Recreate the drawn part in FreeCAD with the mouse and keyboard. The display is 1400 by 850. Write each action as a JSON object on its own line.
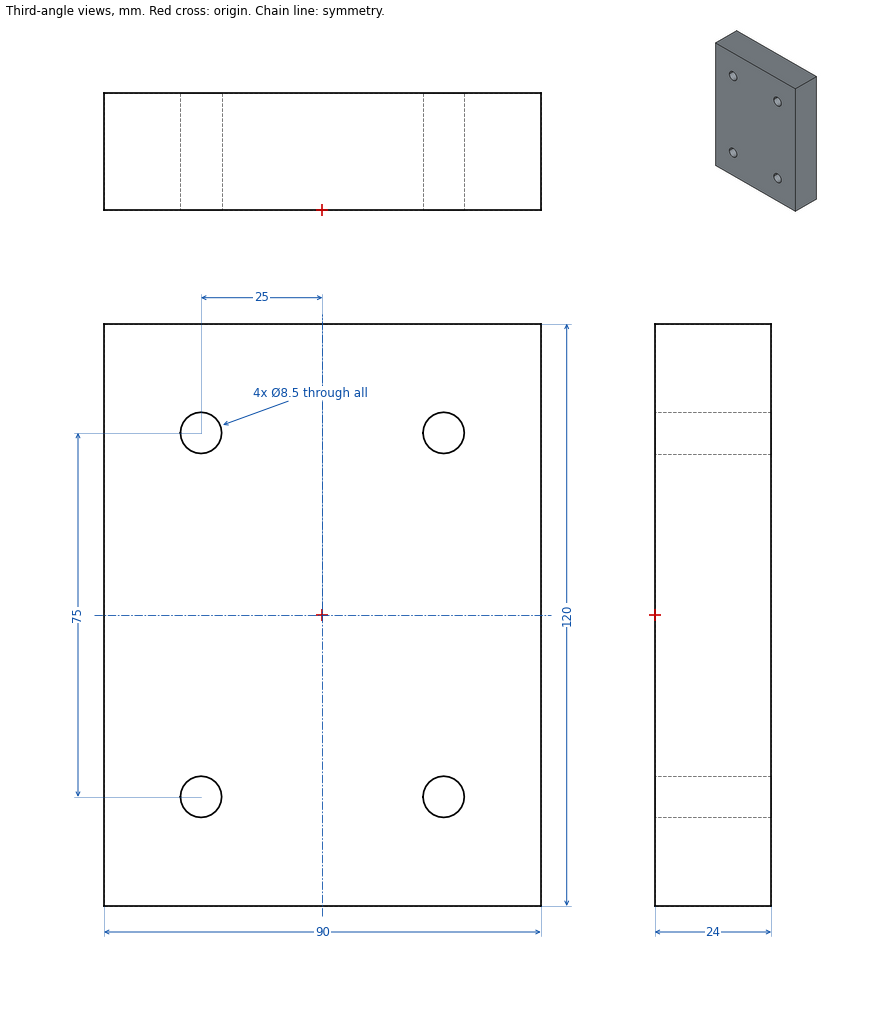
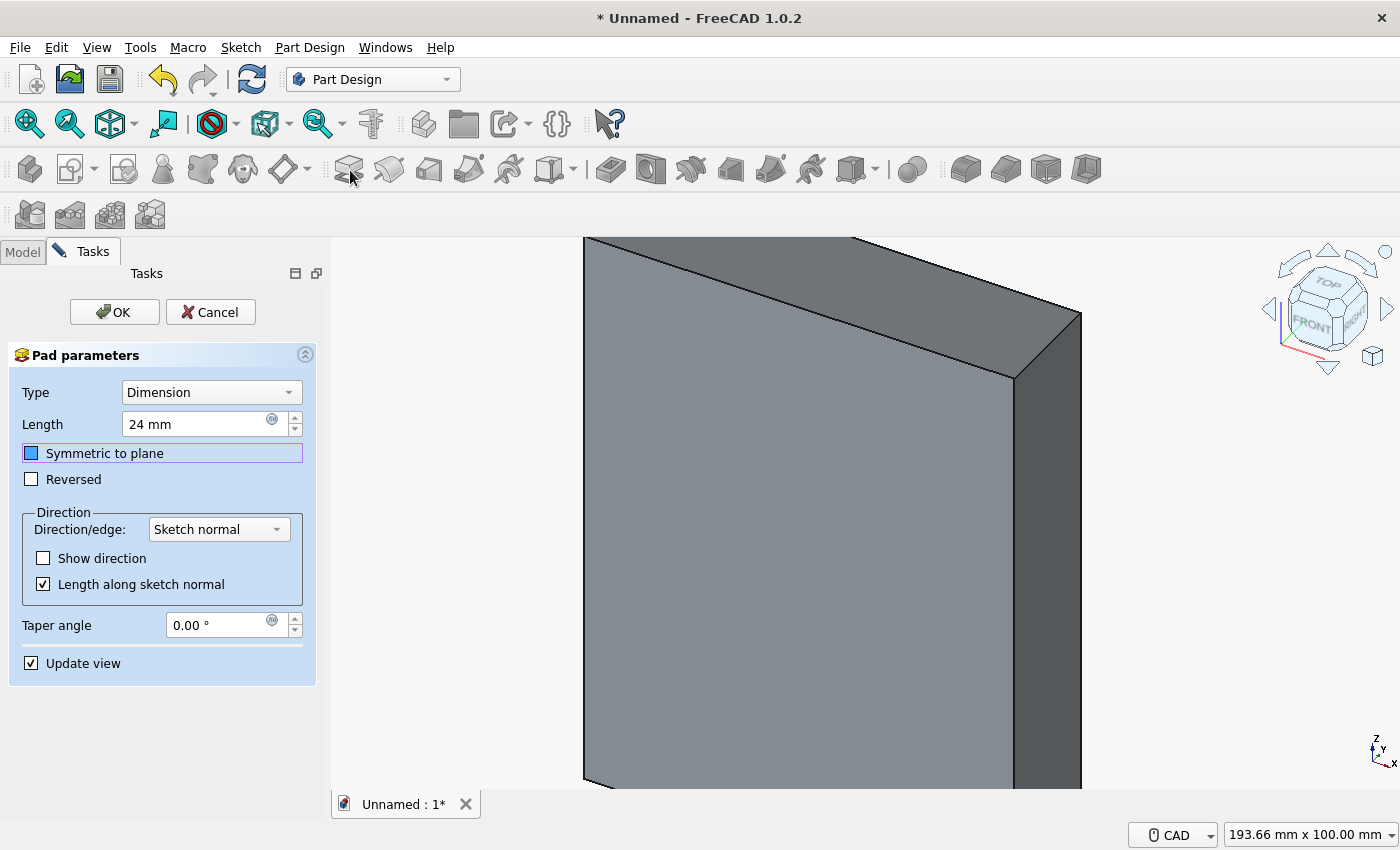
{"action": "left_click", "coordinate": [30, 479]}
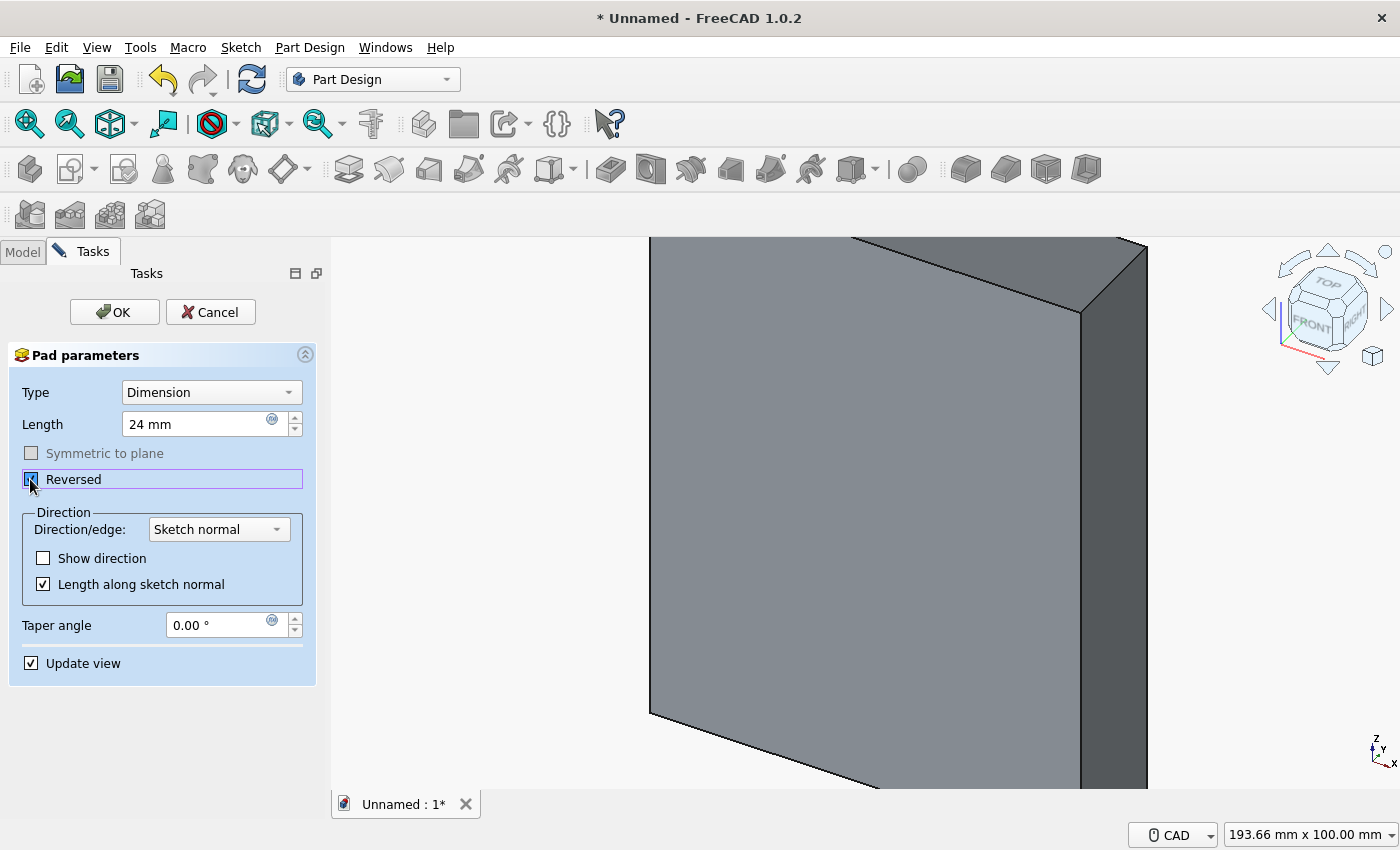
{"action": "left_click", "coordinate": [115, 312]}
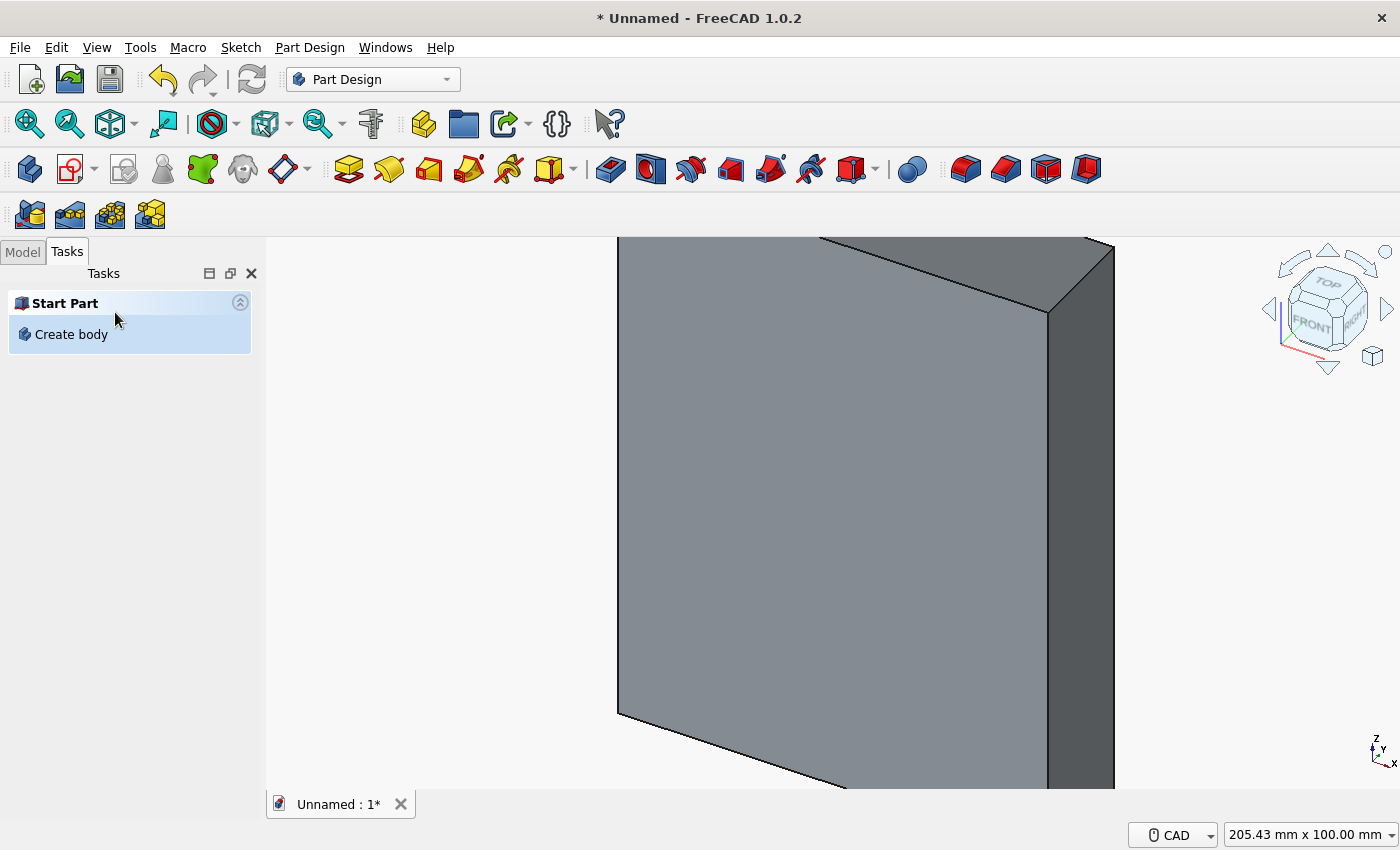
{"action": "left_click", "coordinate": [30, 124]}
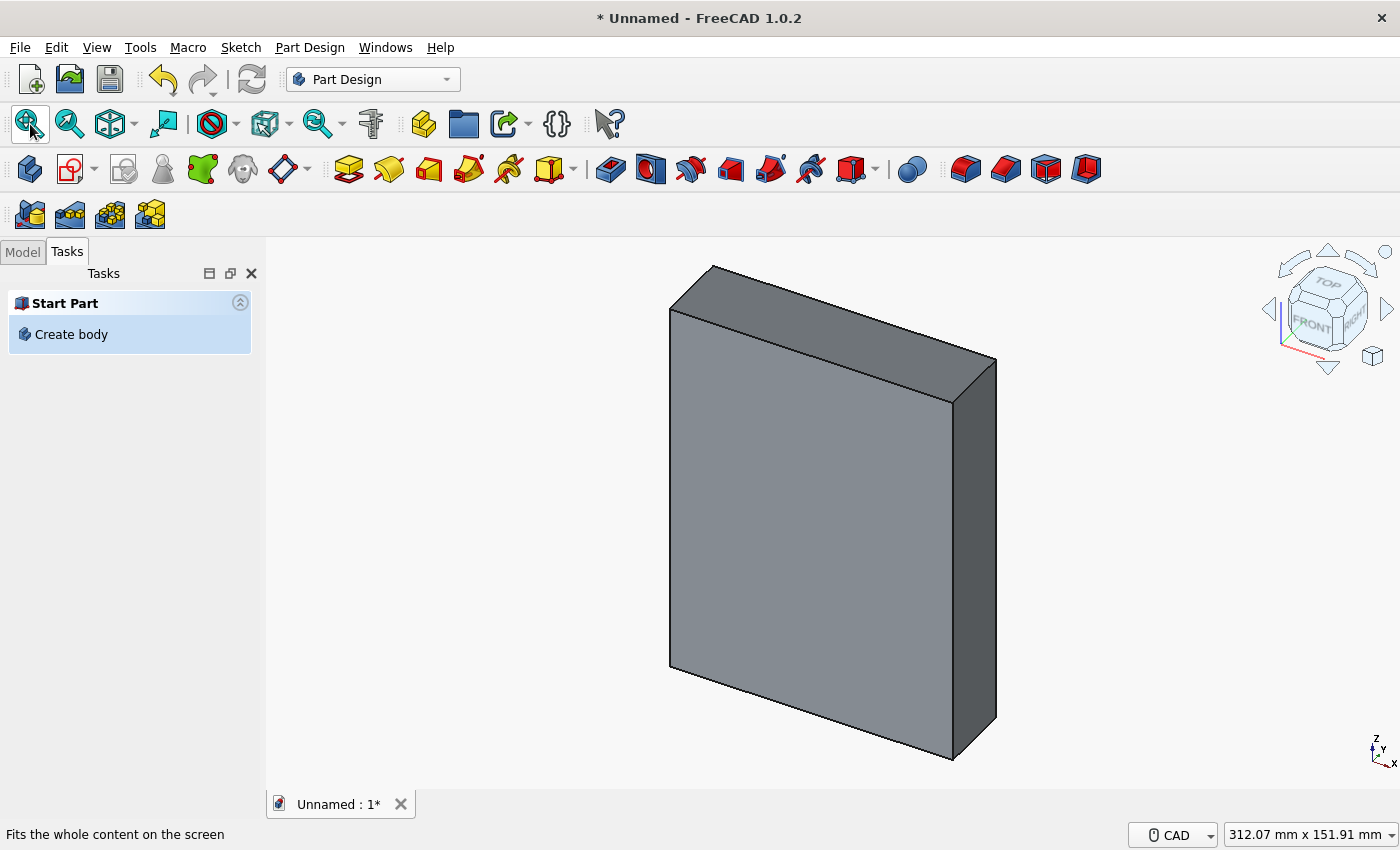
{"action": "key", "text": "4"}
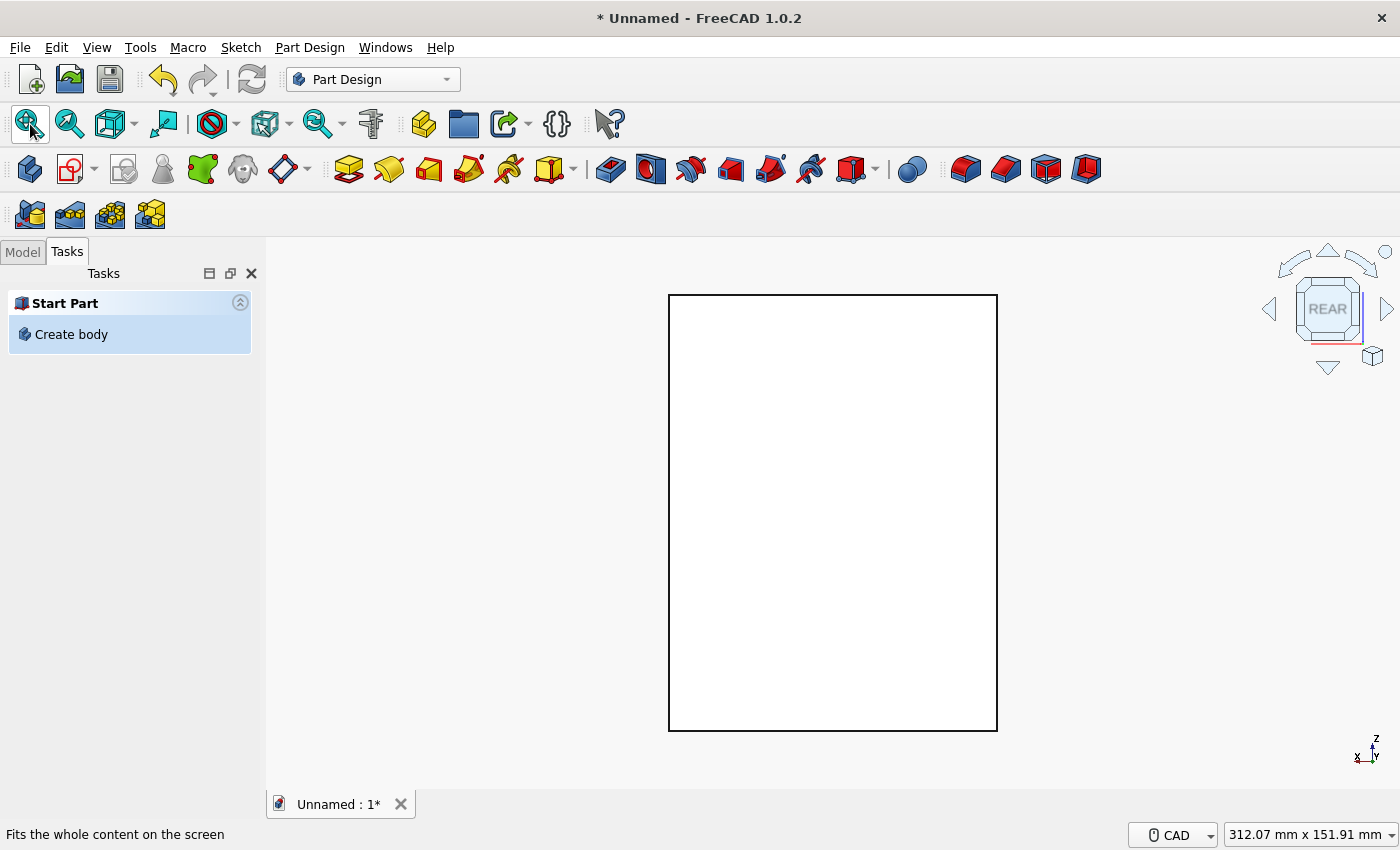
{"action": "left_click", "coordinate": [833, 512]}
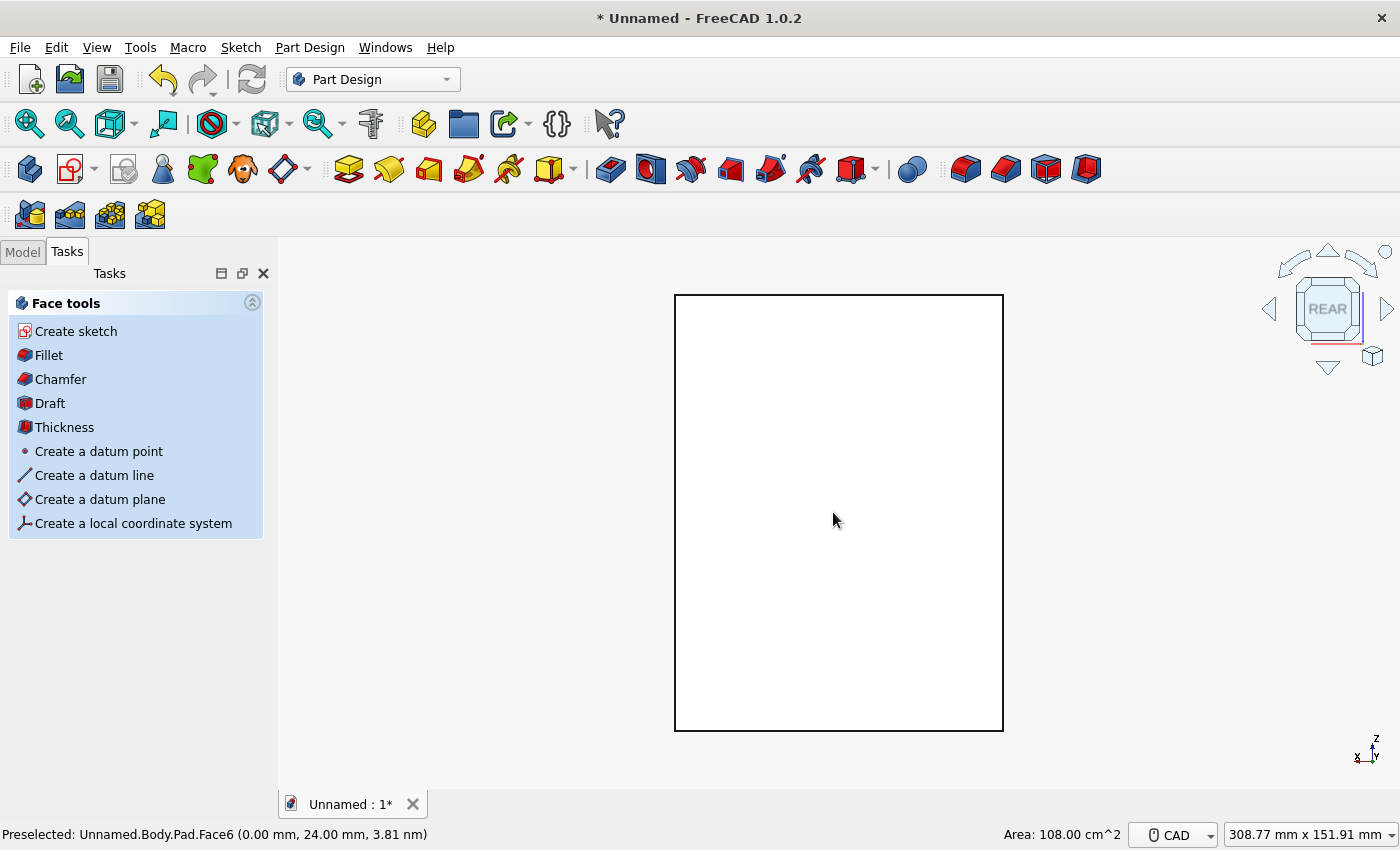
{"action": "left_click", "coordinate": [70, 170]}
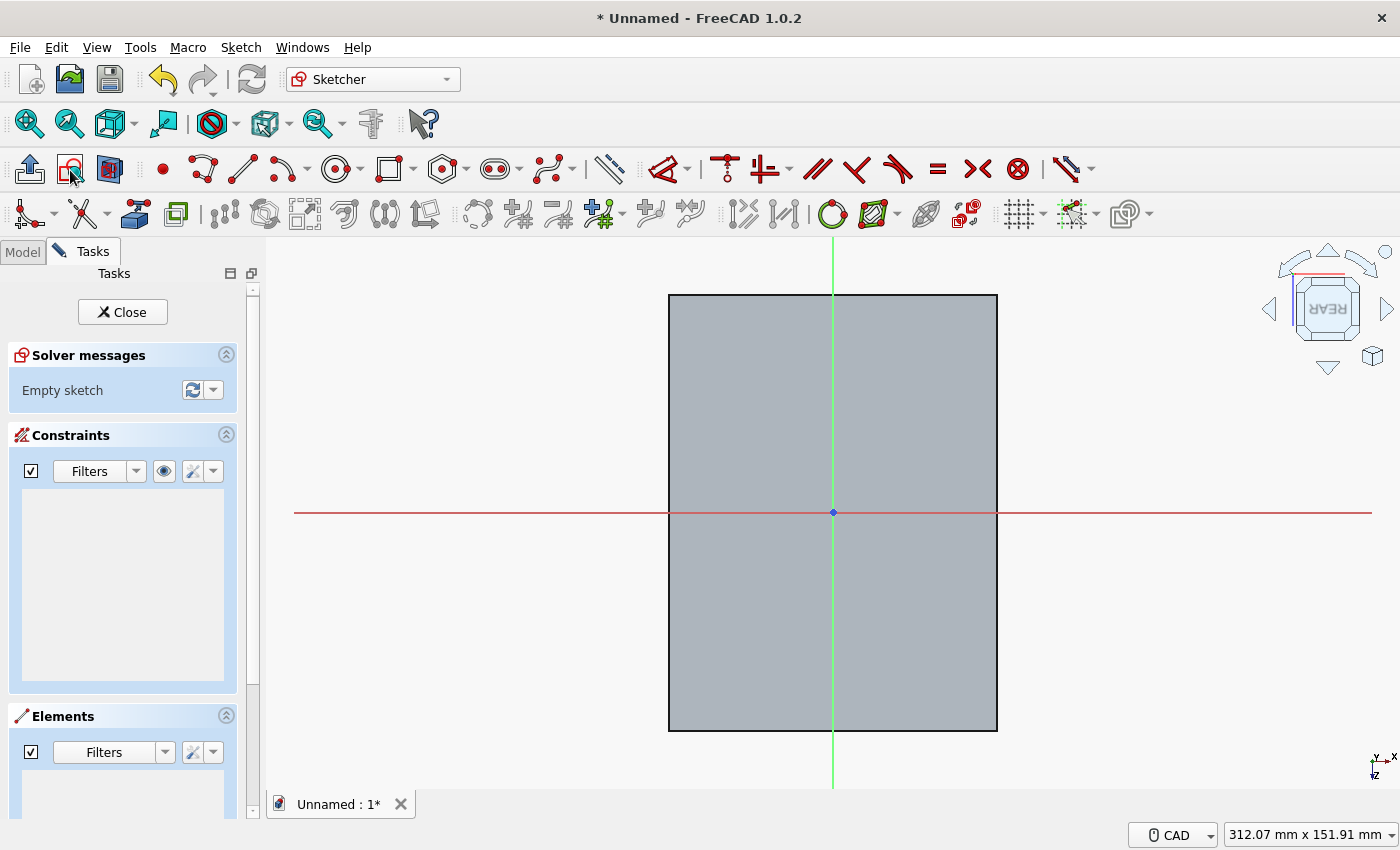
{"action": "key", "text": "g c"}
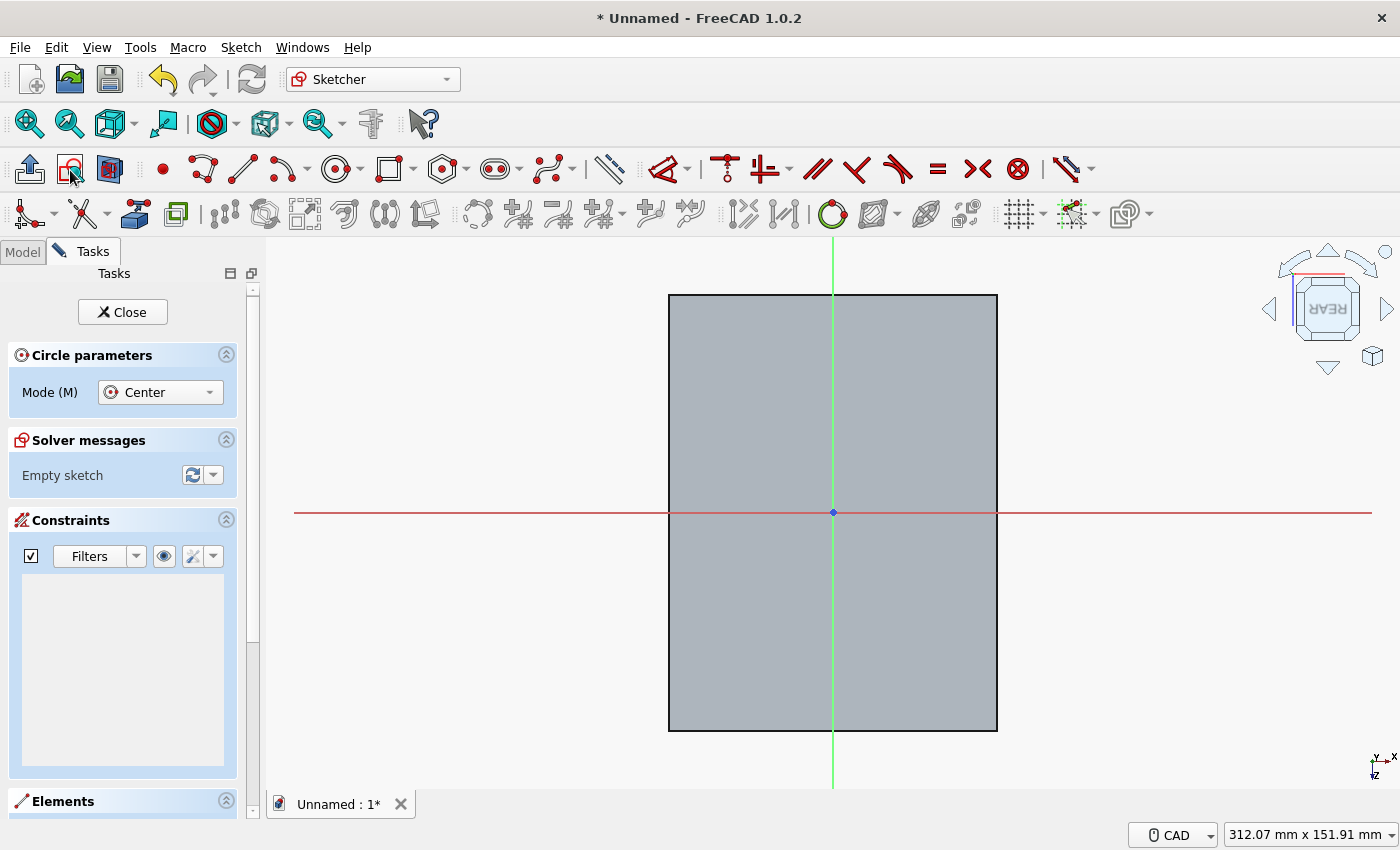
{"action": "scroll", "coordinate": [742, 649], "scroll_direction": "up", "scroll_amount": 2}